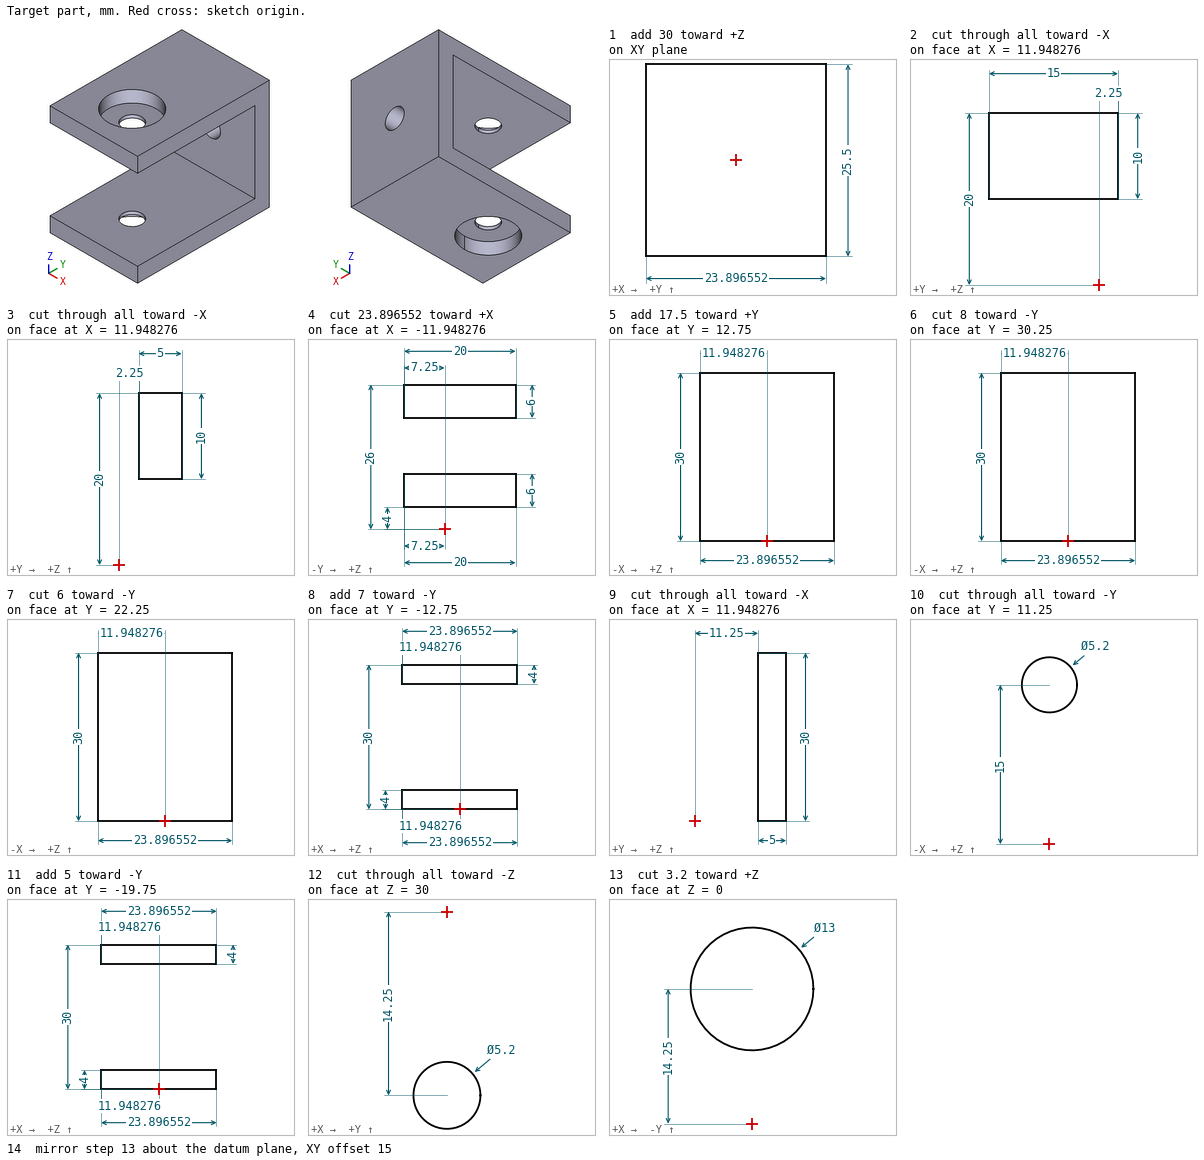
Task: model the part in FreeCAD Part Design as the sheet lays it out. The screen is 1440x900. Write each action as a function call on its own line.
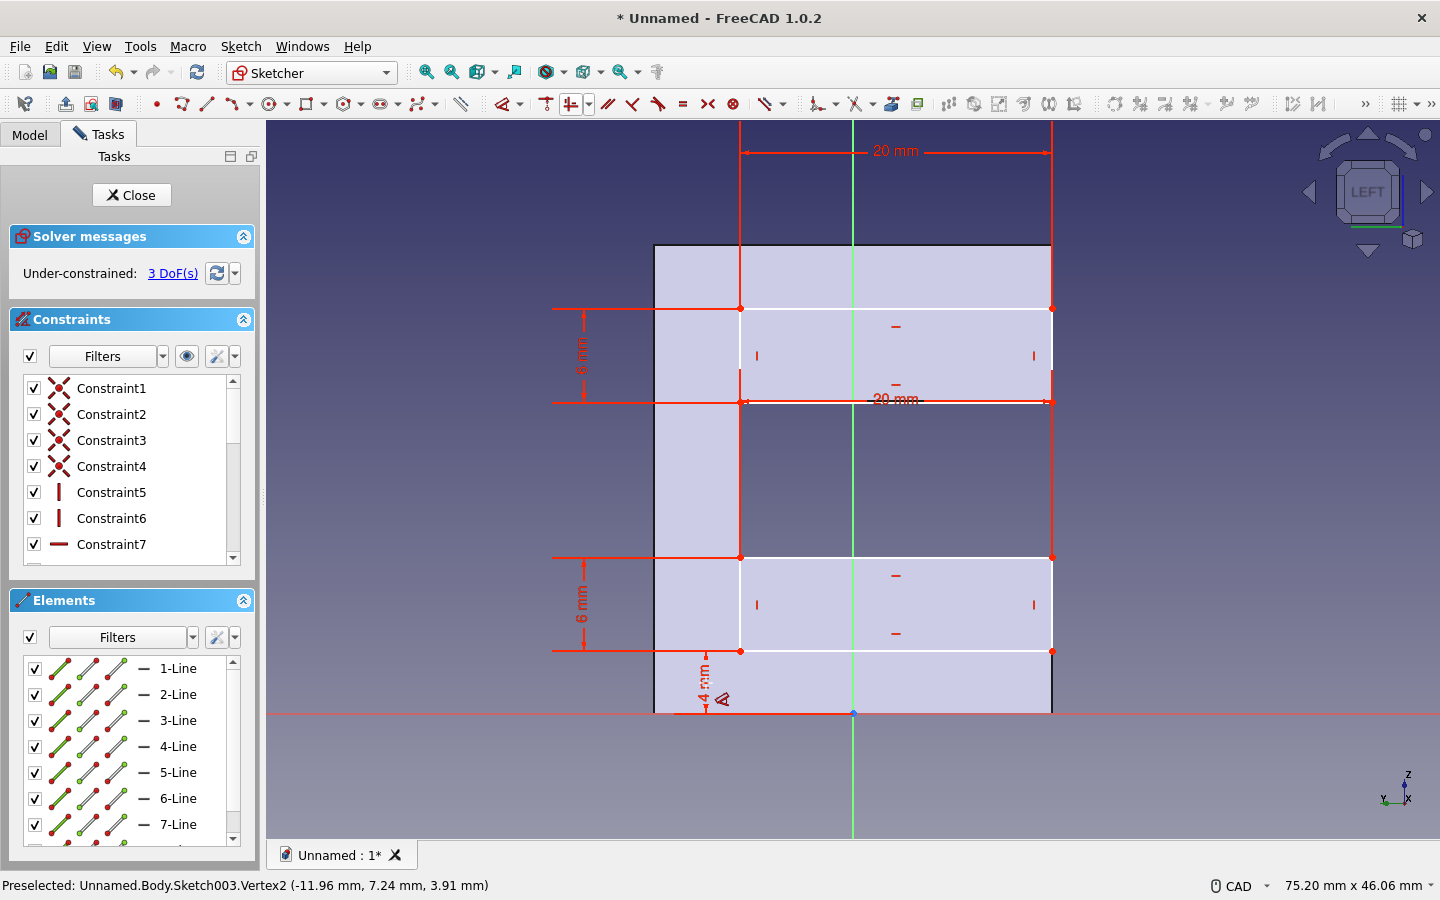
click(740, 309)
click(706, 511)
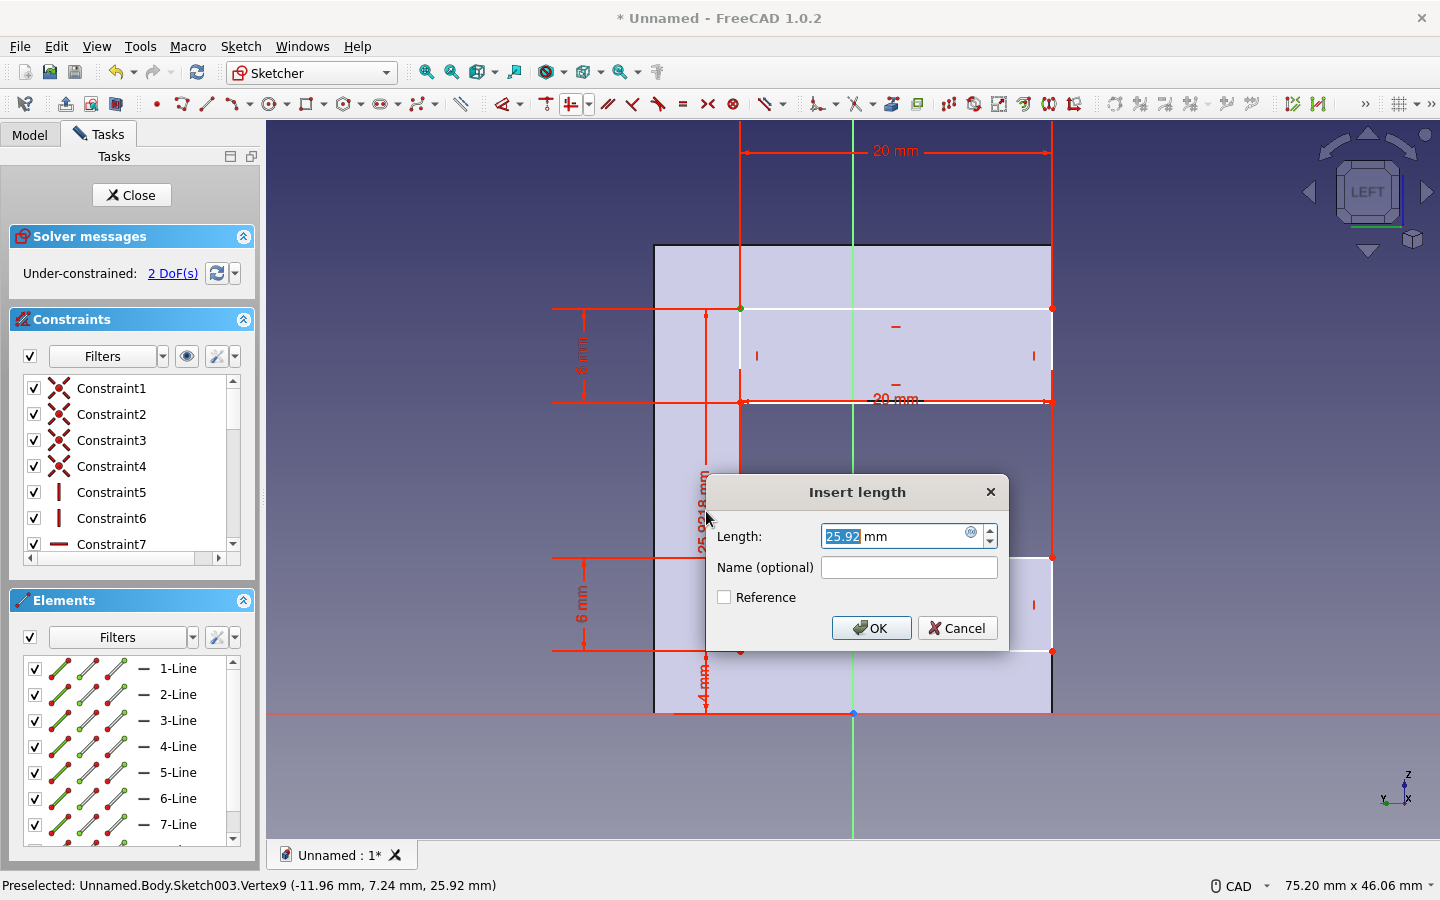
text(26)
key(Return)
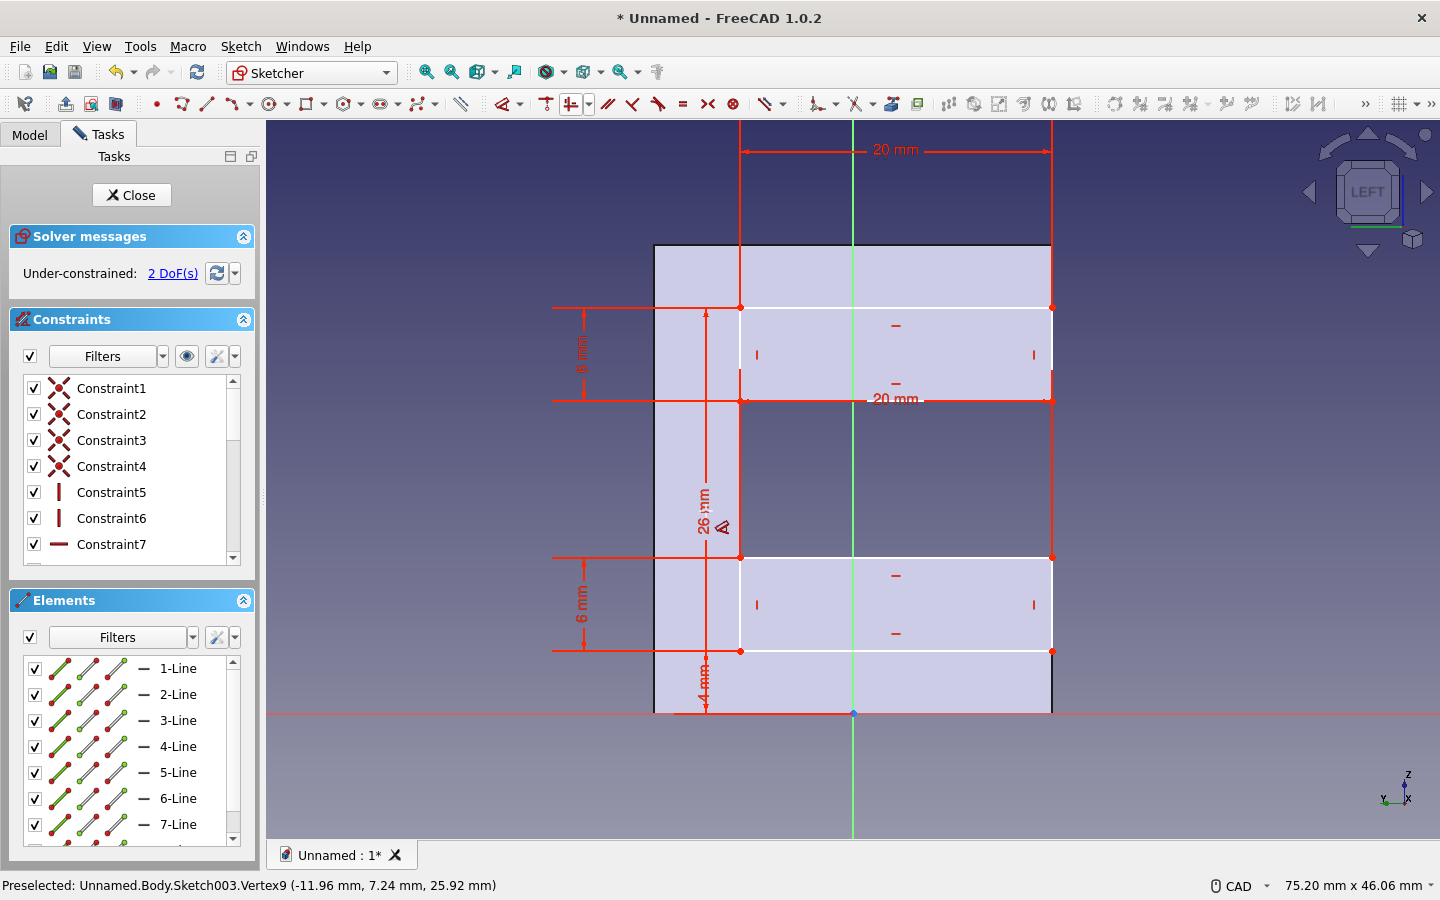
click(740, 558)
click(796, 748)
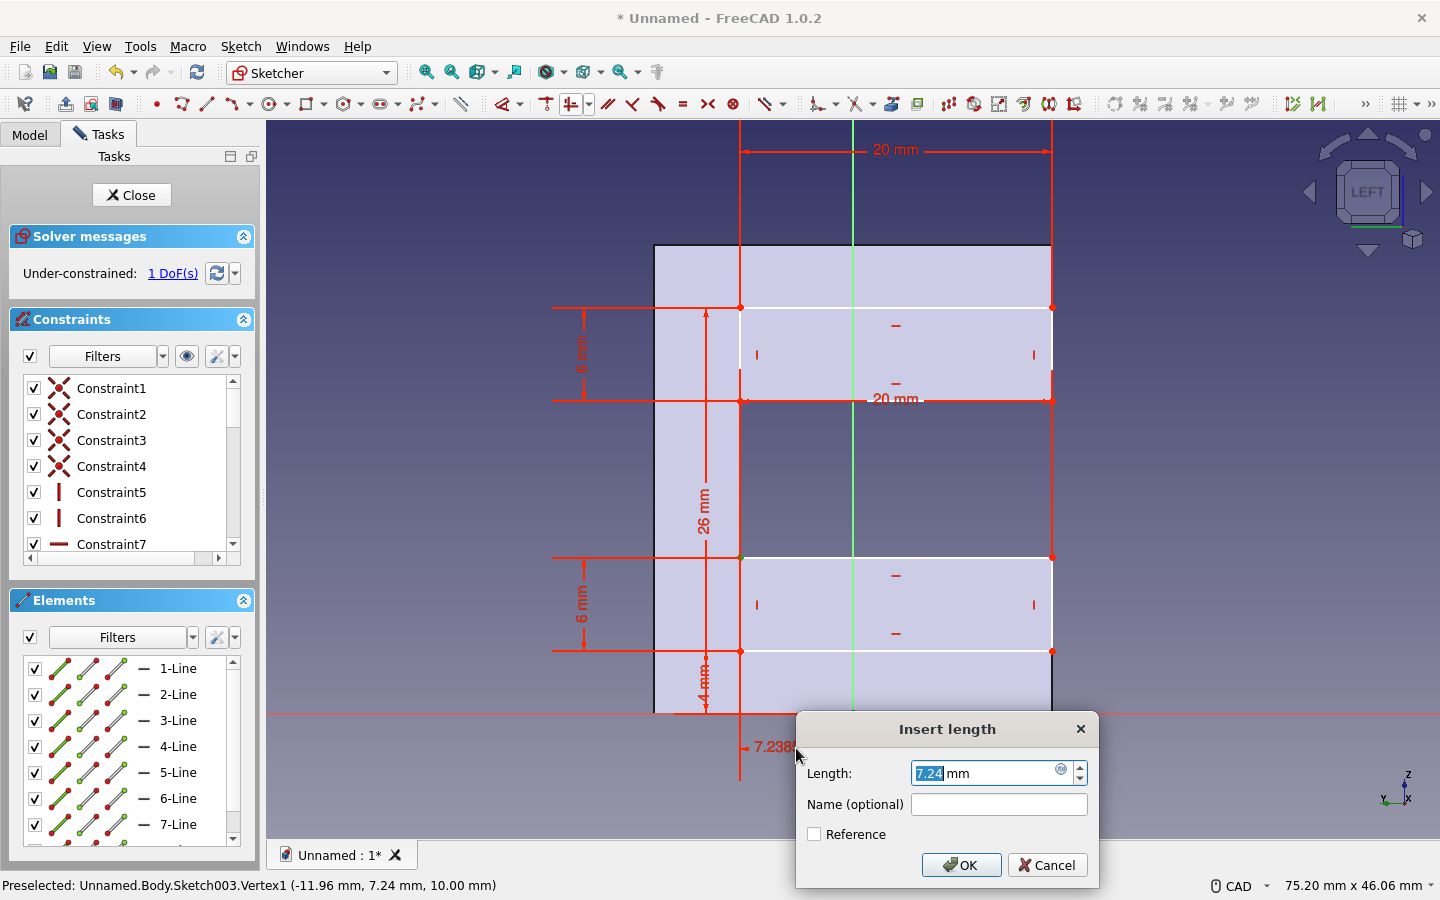
text(7.25)
key(Return)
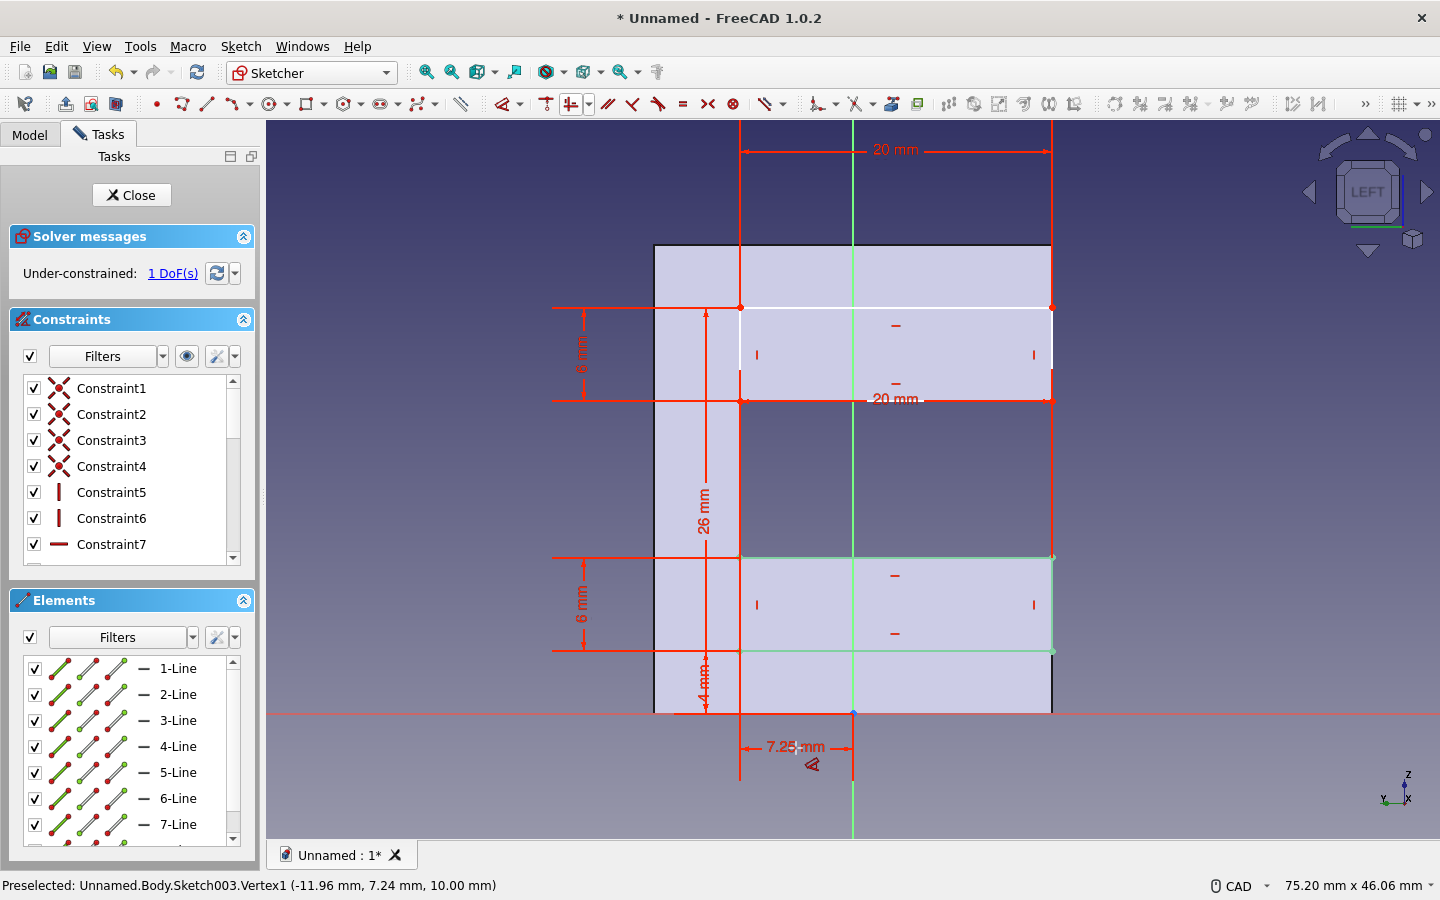
click(740, 308)
click(796, 274)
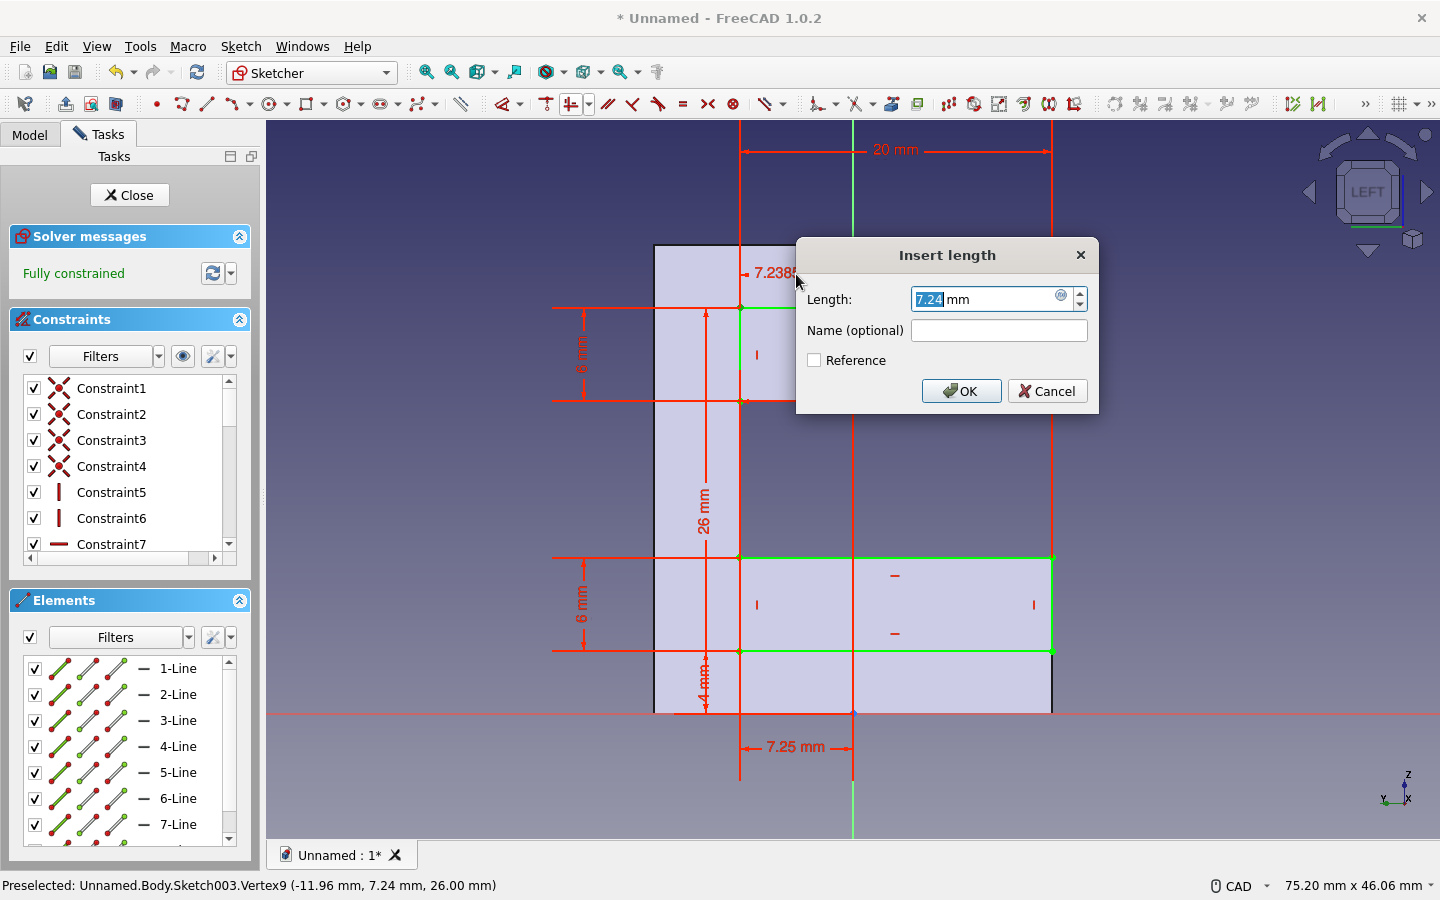
text(7.25)
key(Return)
key(Escape)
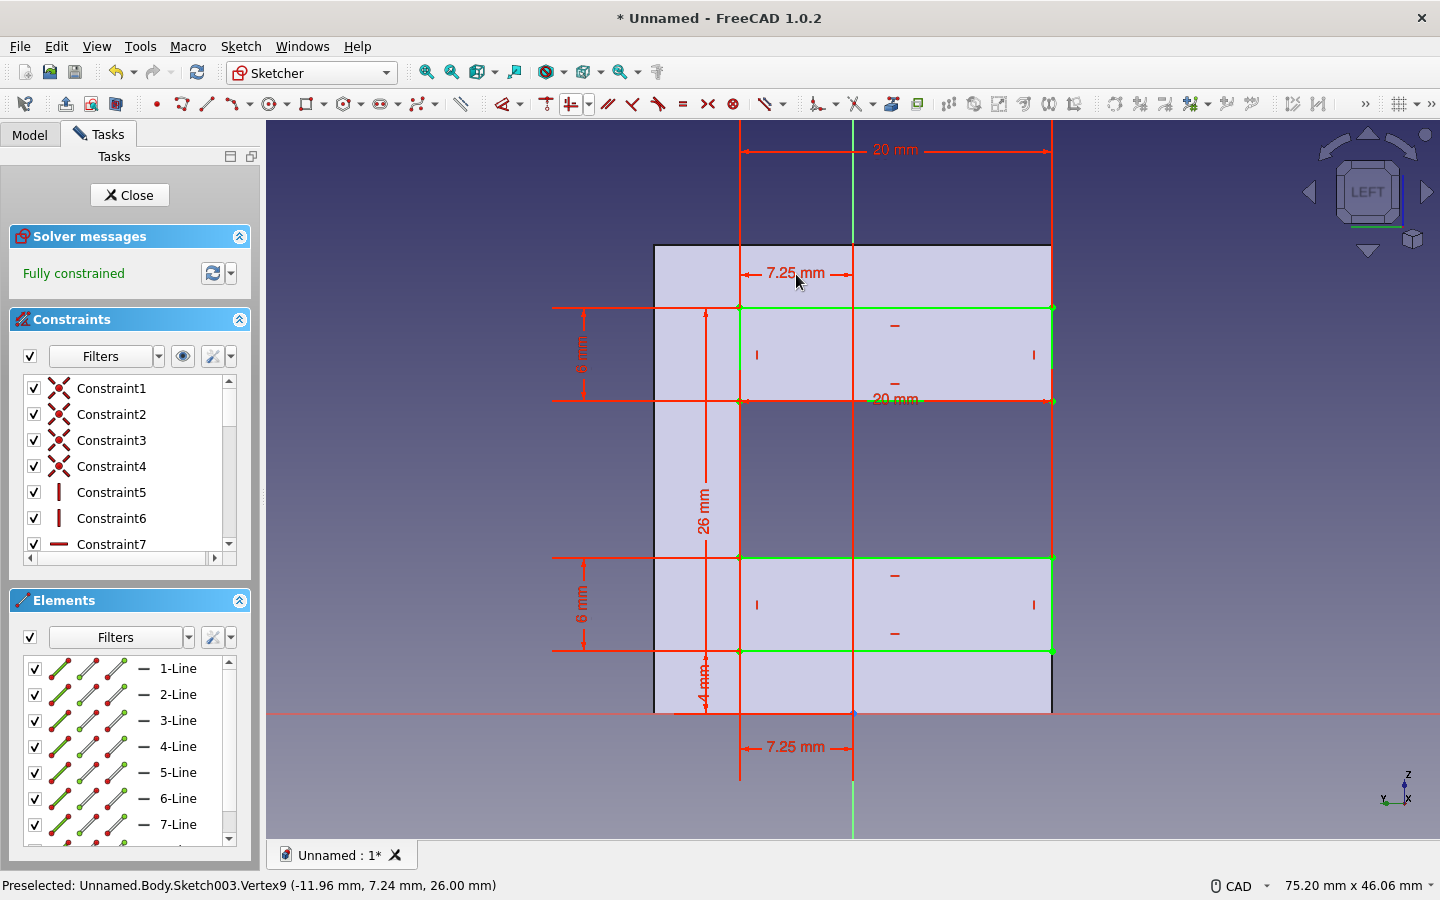
click(130, 195)